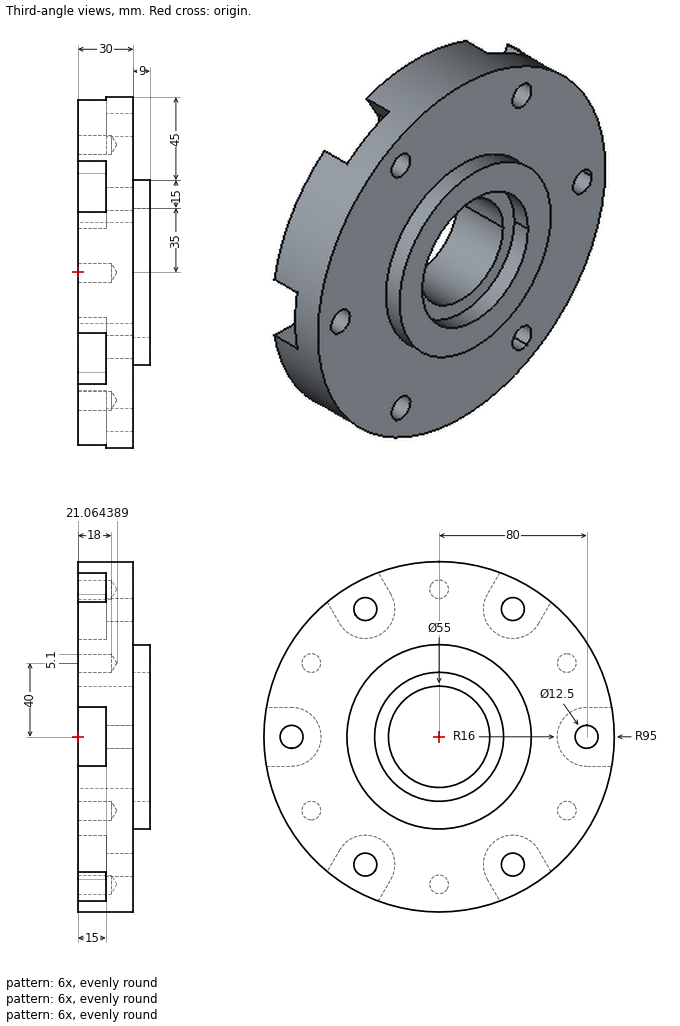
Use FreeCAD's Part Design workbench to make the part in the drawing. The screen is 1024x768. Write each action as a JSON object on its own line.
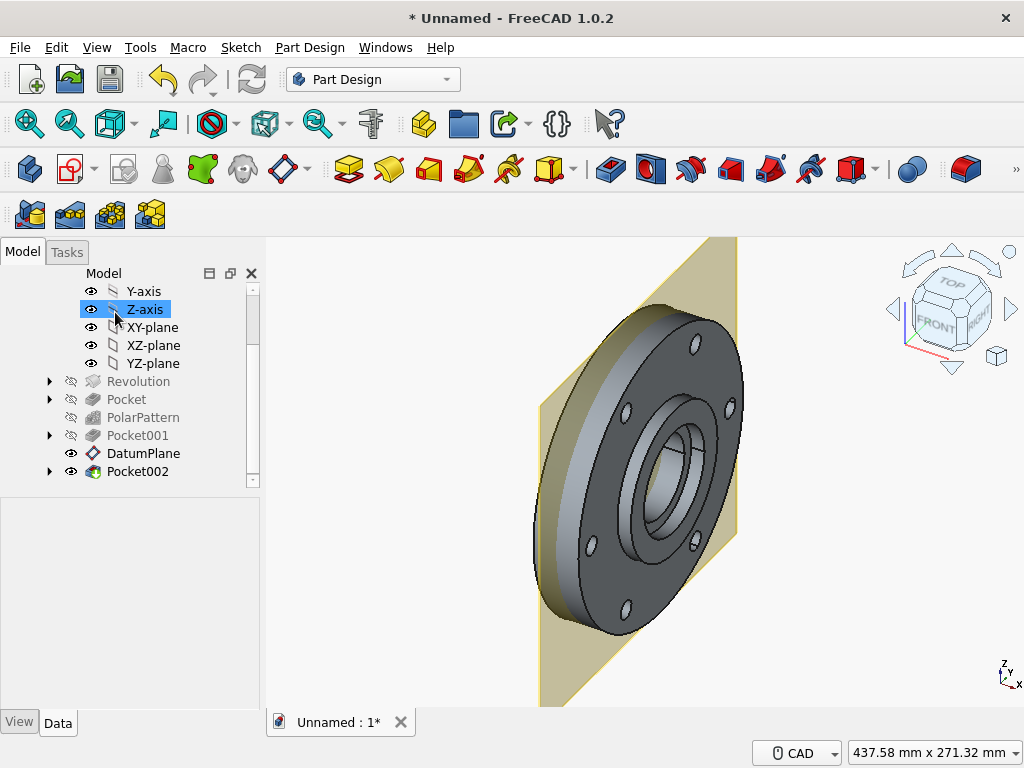
{"action": "left_click", "coordinate": [116, 453]}
{"action": "key", "text": "space"}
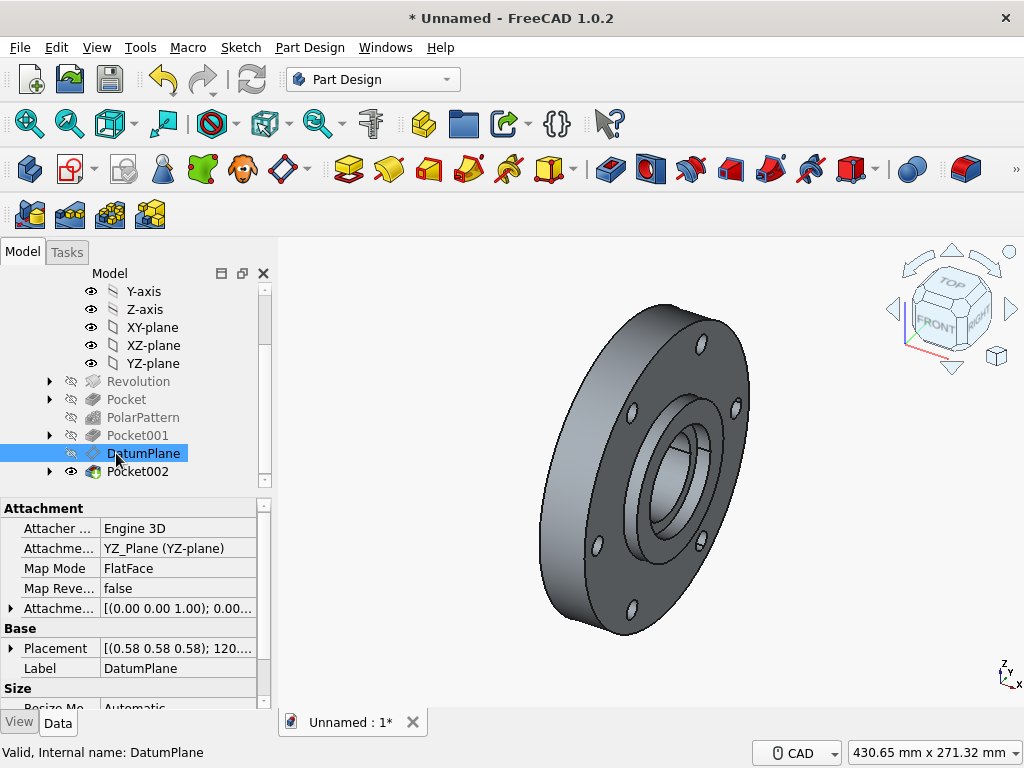
{"action": "left_click", "coordinate": [116, 471]}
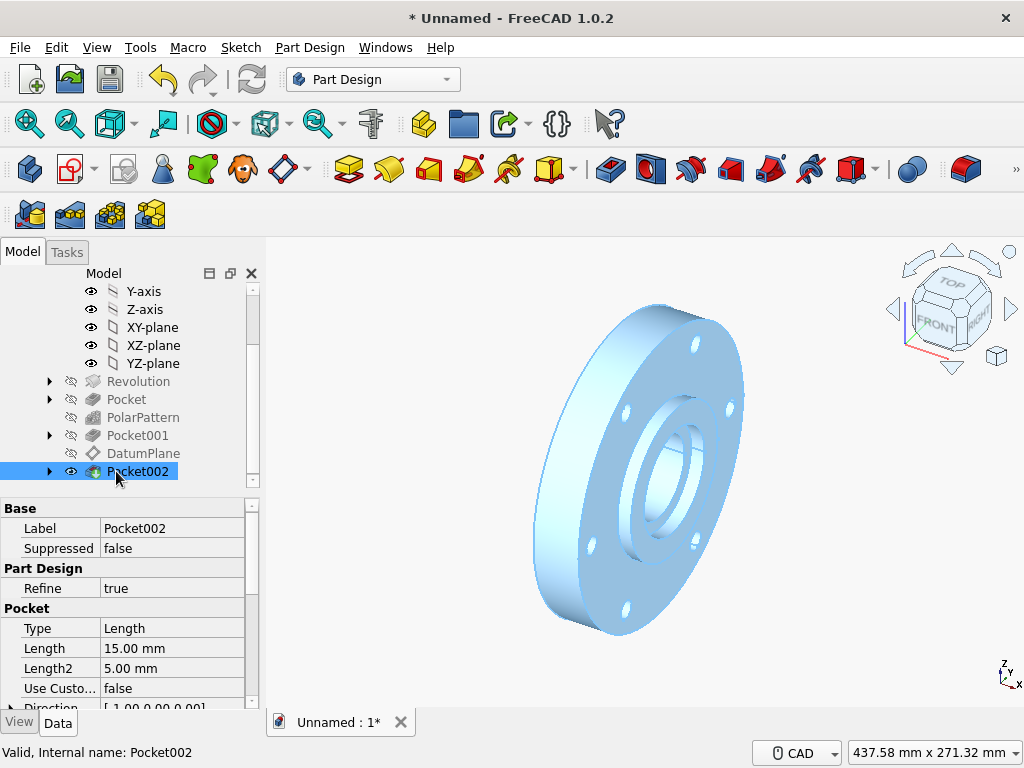
{"action": "left_click", "coordinate": [110, 214]}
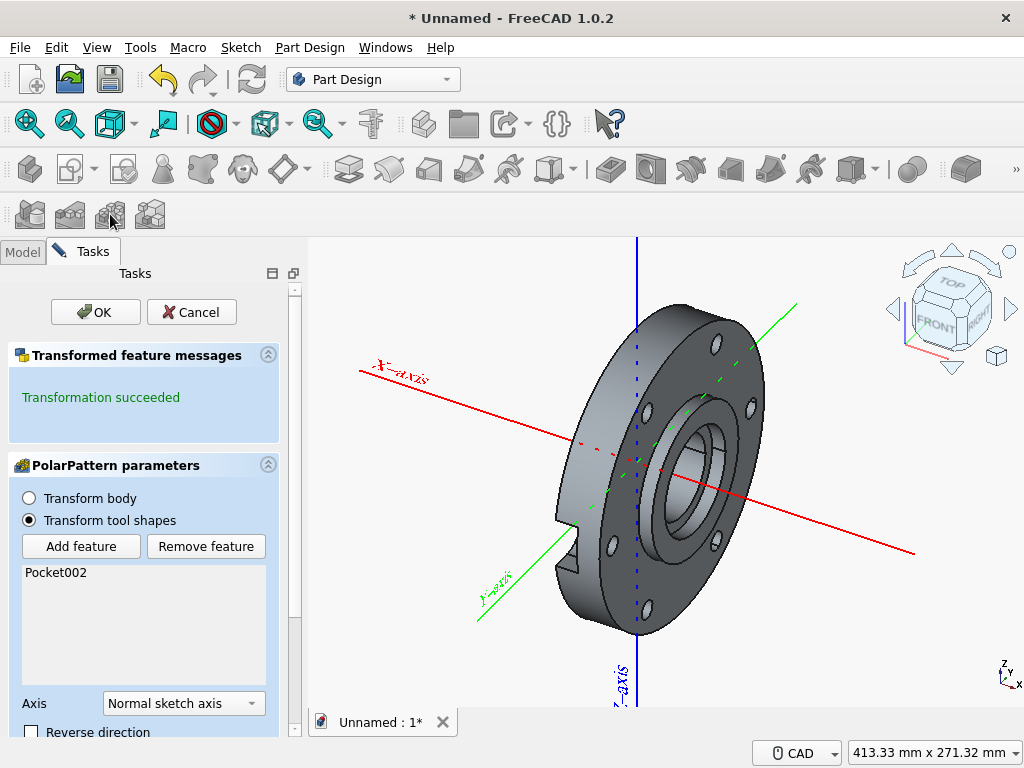
{"action": "left_click", "coordinate": [184, 704]}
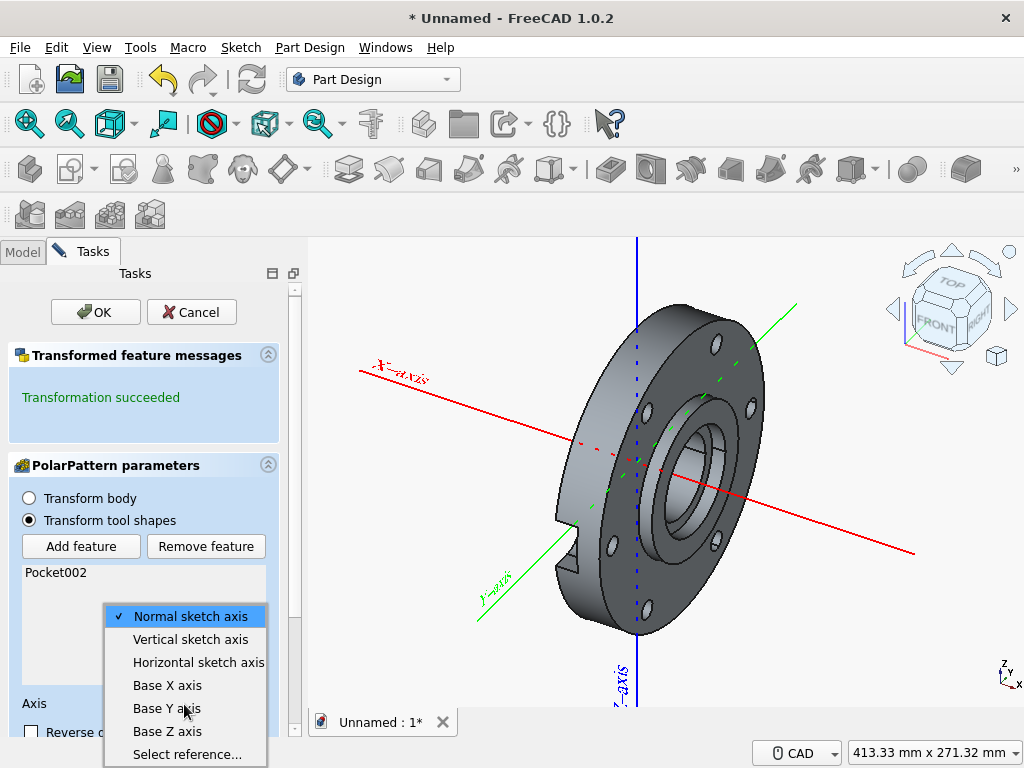
{"action": "left_click", "coordinate": [184, 686]}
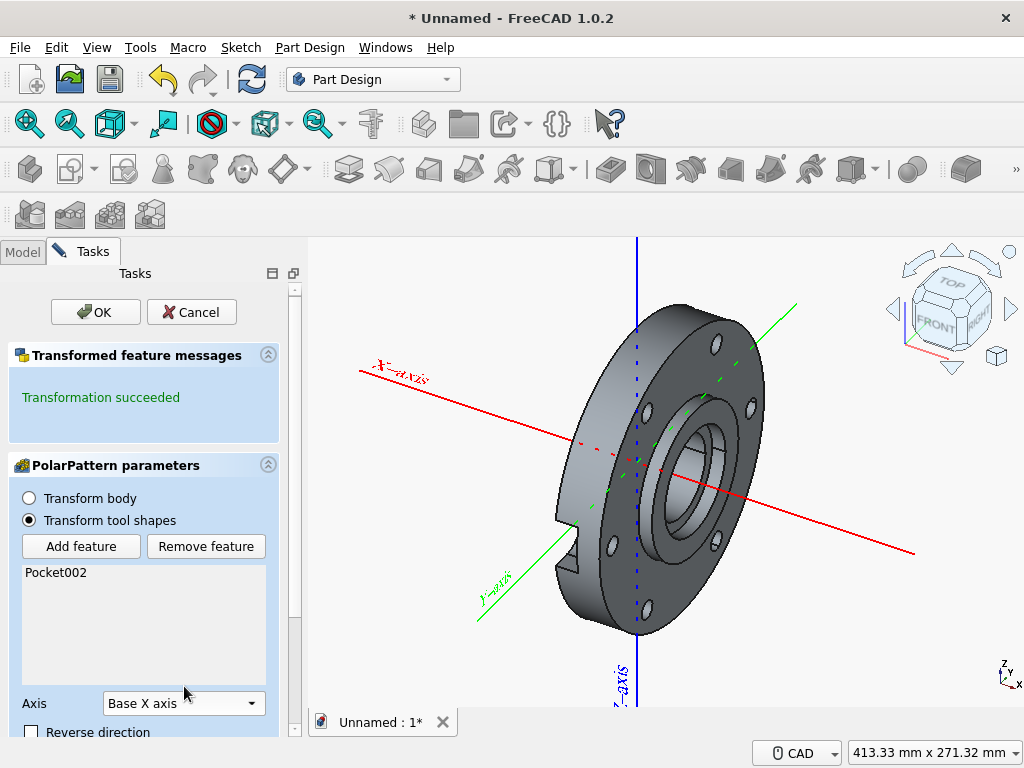
{"action": "scroll", "coordinate": [295, 510], "scroll_direction": "down", "scroll_amount": 3}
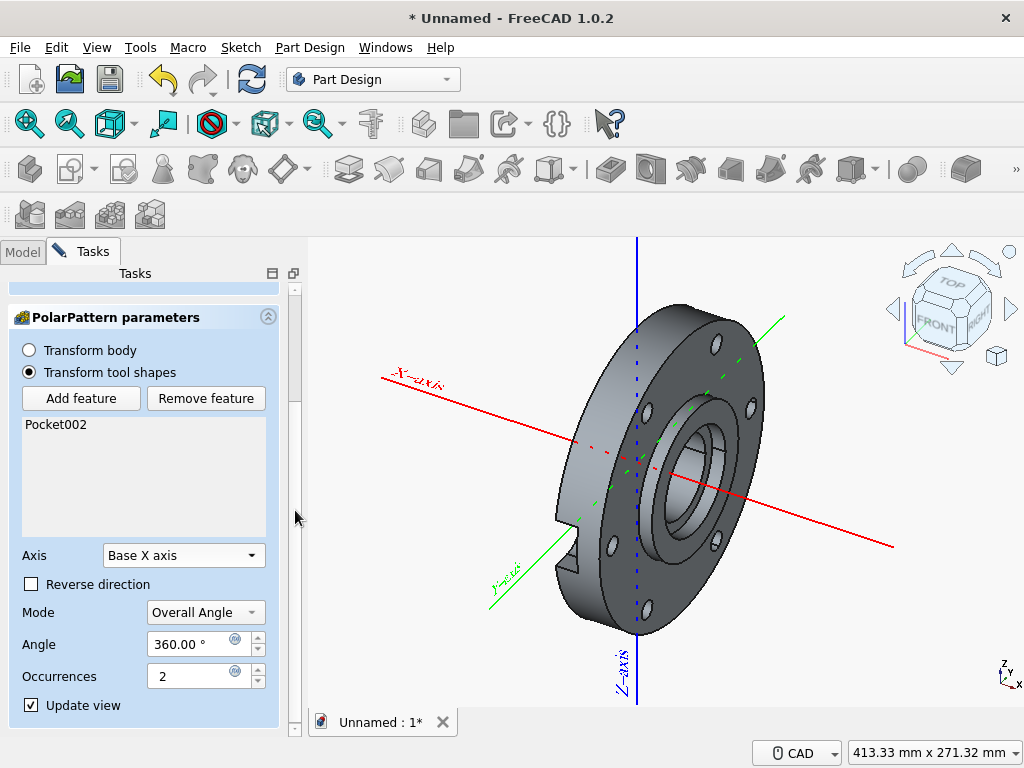
{"action": "triple_click", "coordinate": [198, 676]}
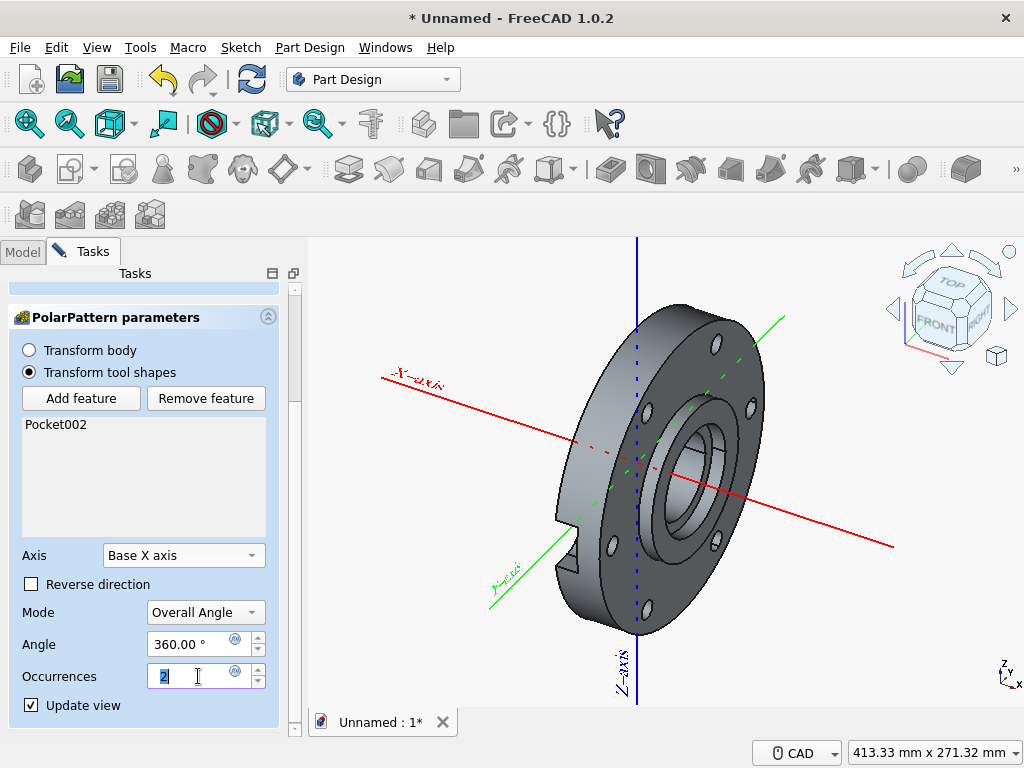
{"action": "type", "text": "6"}
{"action": "key", "text": "Tab"}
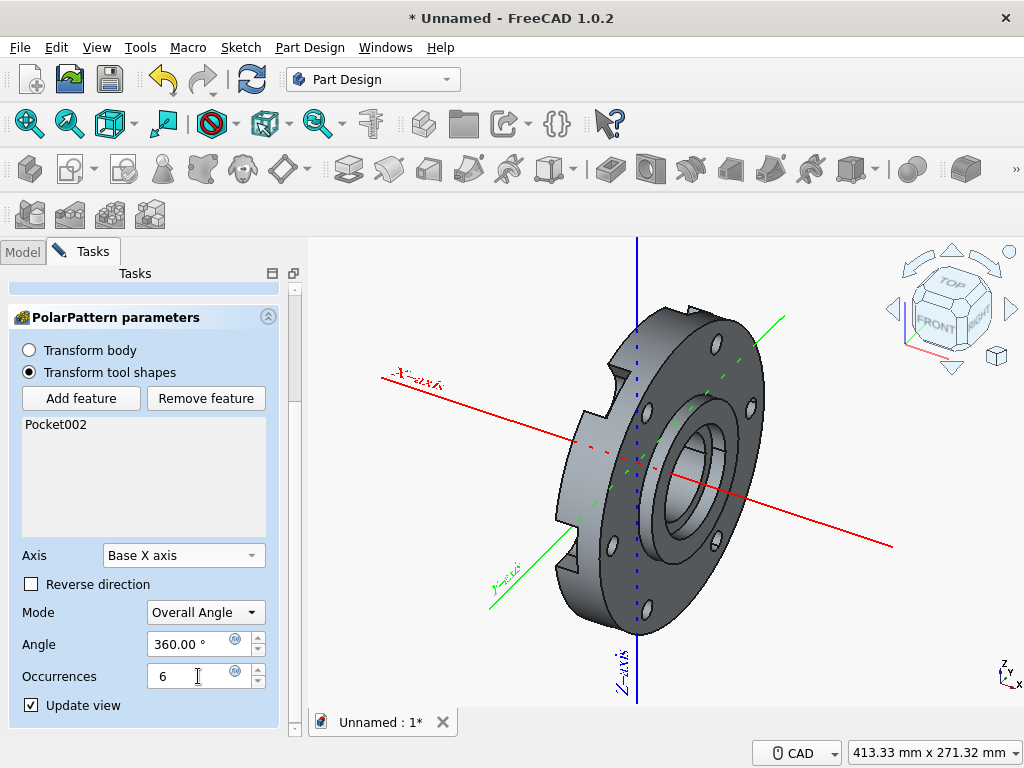
{"action": "scroll", "coordinate": [295, 510], "scroll_direction": "up", "scroll_amount": 4}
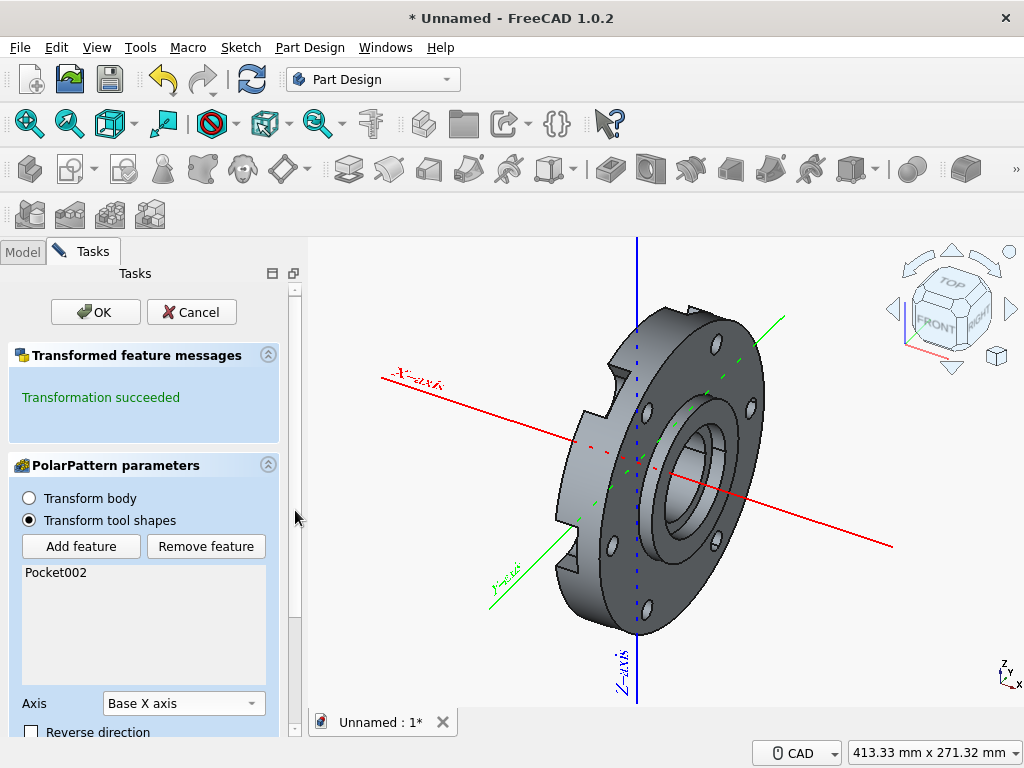
{"action": "left_click", "coordinate": [96, 312]}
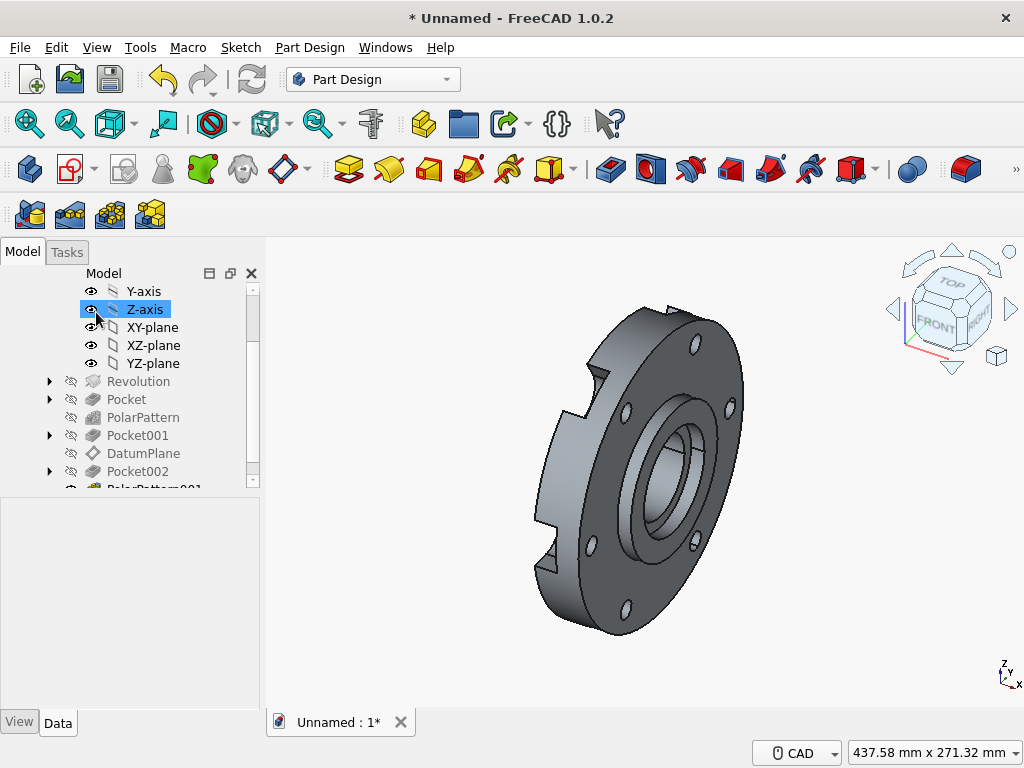
{"action": "scroll", "coordinate": [160, 377], "scroll_direction": "down", "scroll_amount": 3}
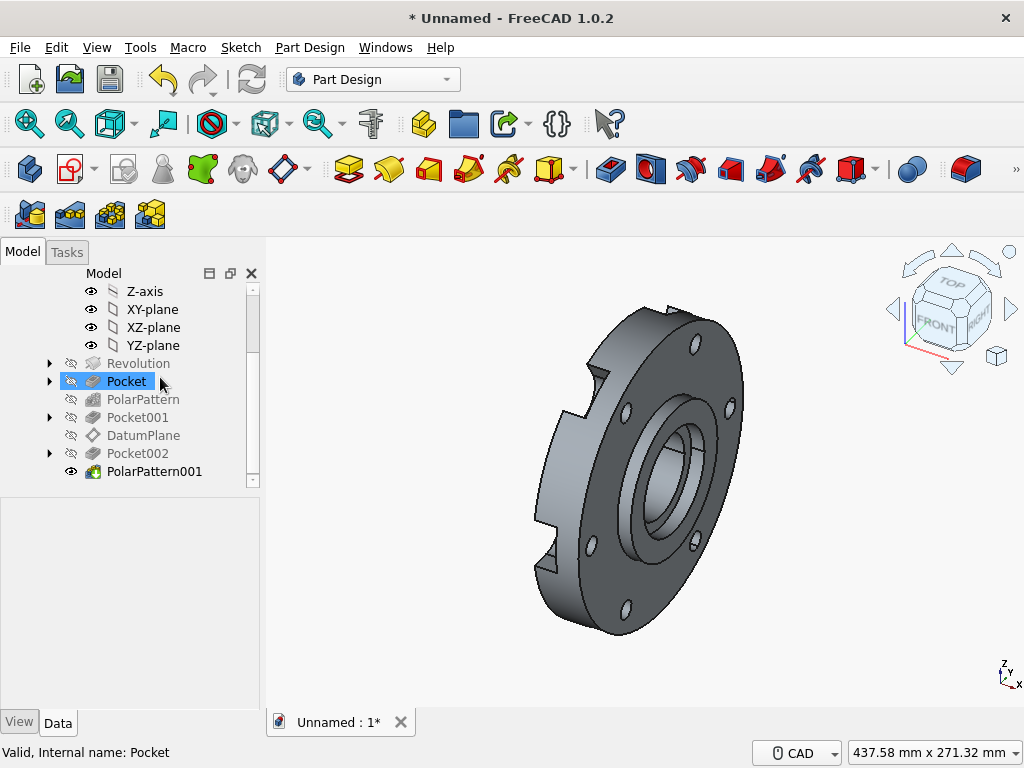
{"action": "scroll", "coordinate": [160, 377], "scroll_direction": "up", "scroll_amount": 15}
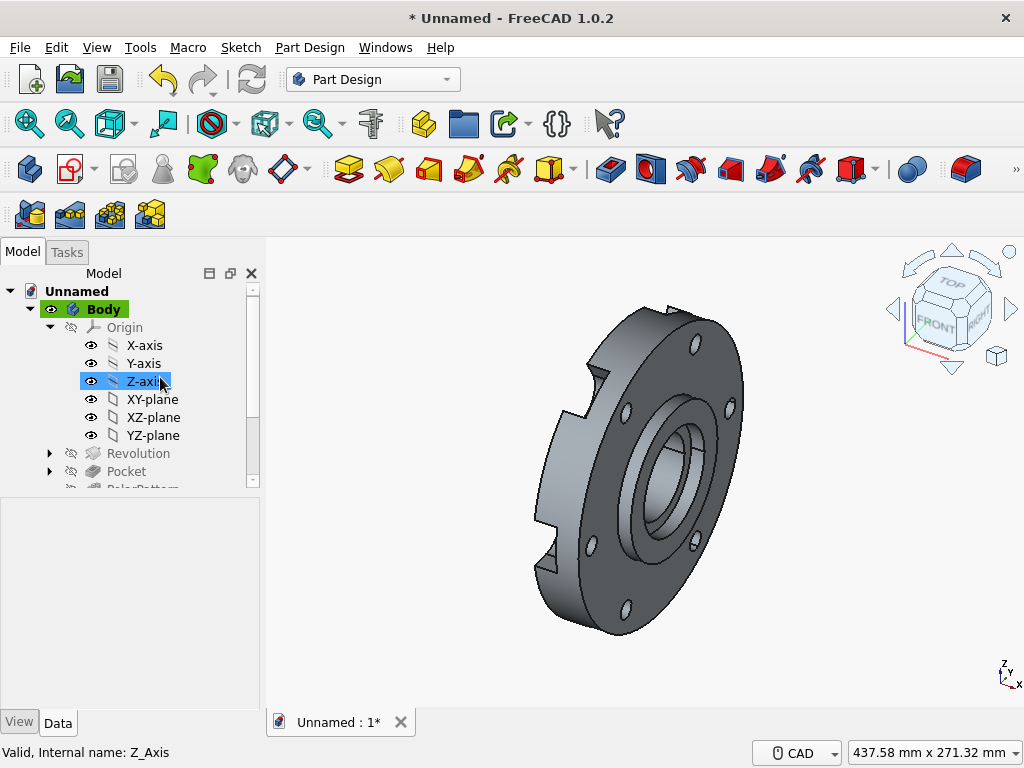
{"action": "left_click", "coordinate": [136, 417]}